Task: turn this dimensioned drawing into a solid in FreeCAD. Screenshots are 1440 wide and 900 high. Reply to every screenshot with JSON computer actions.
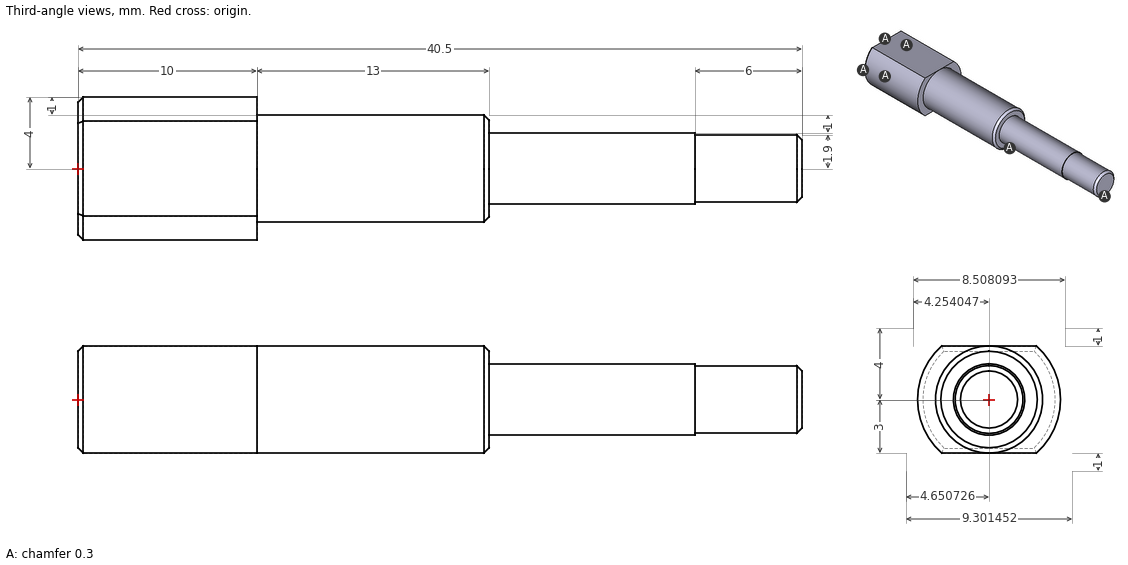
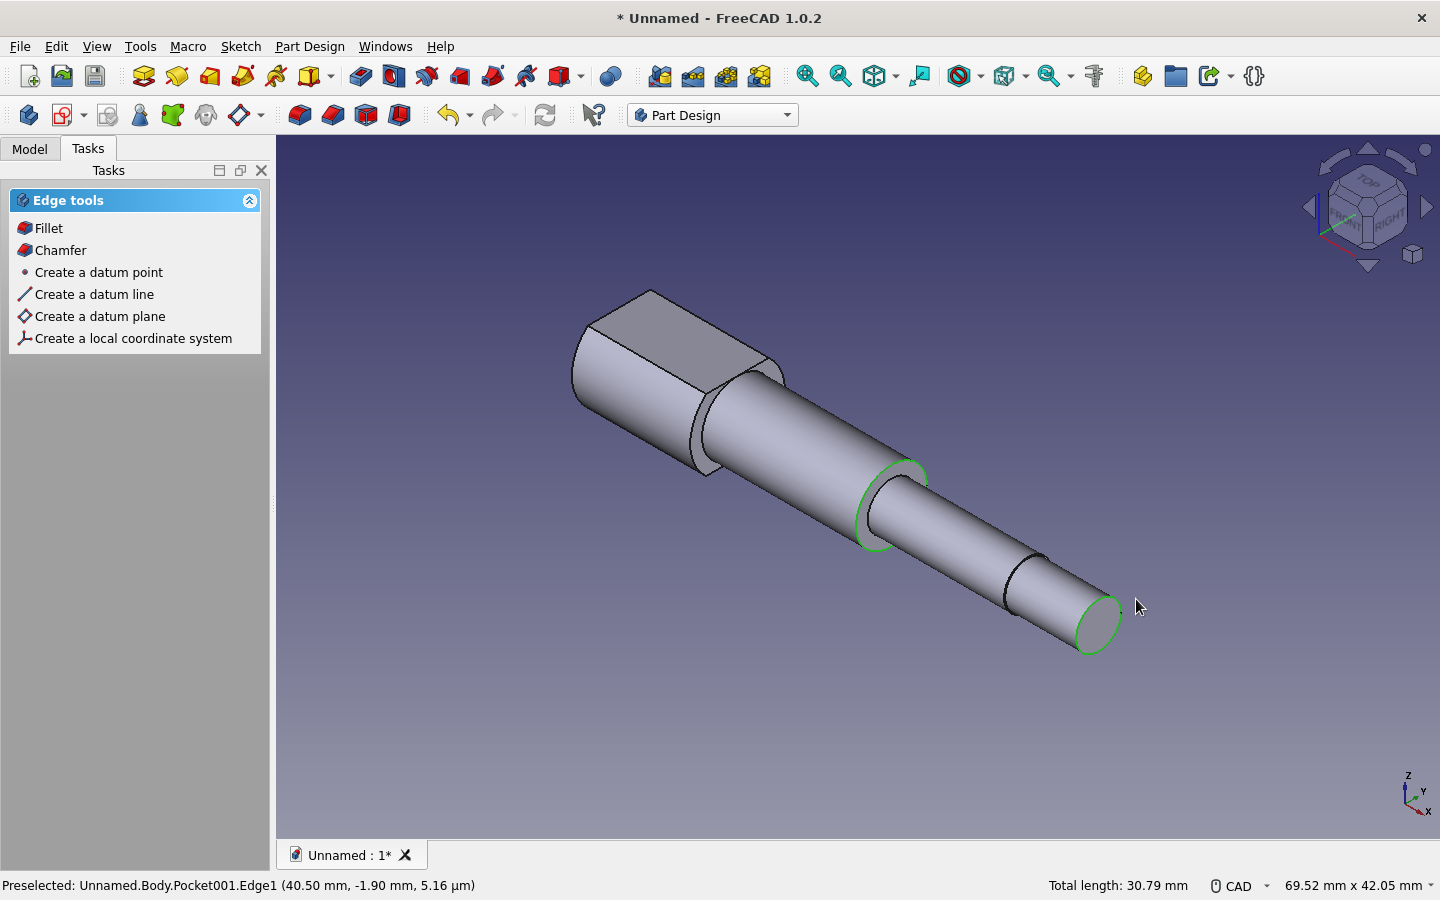
{"action": "left_click", "coordinate": [574, 392], "text": "ctrl"}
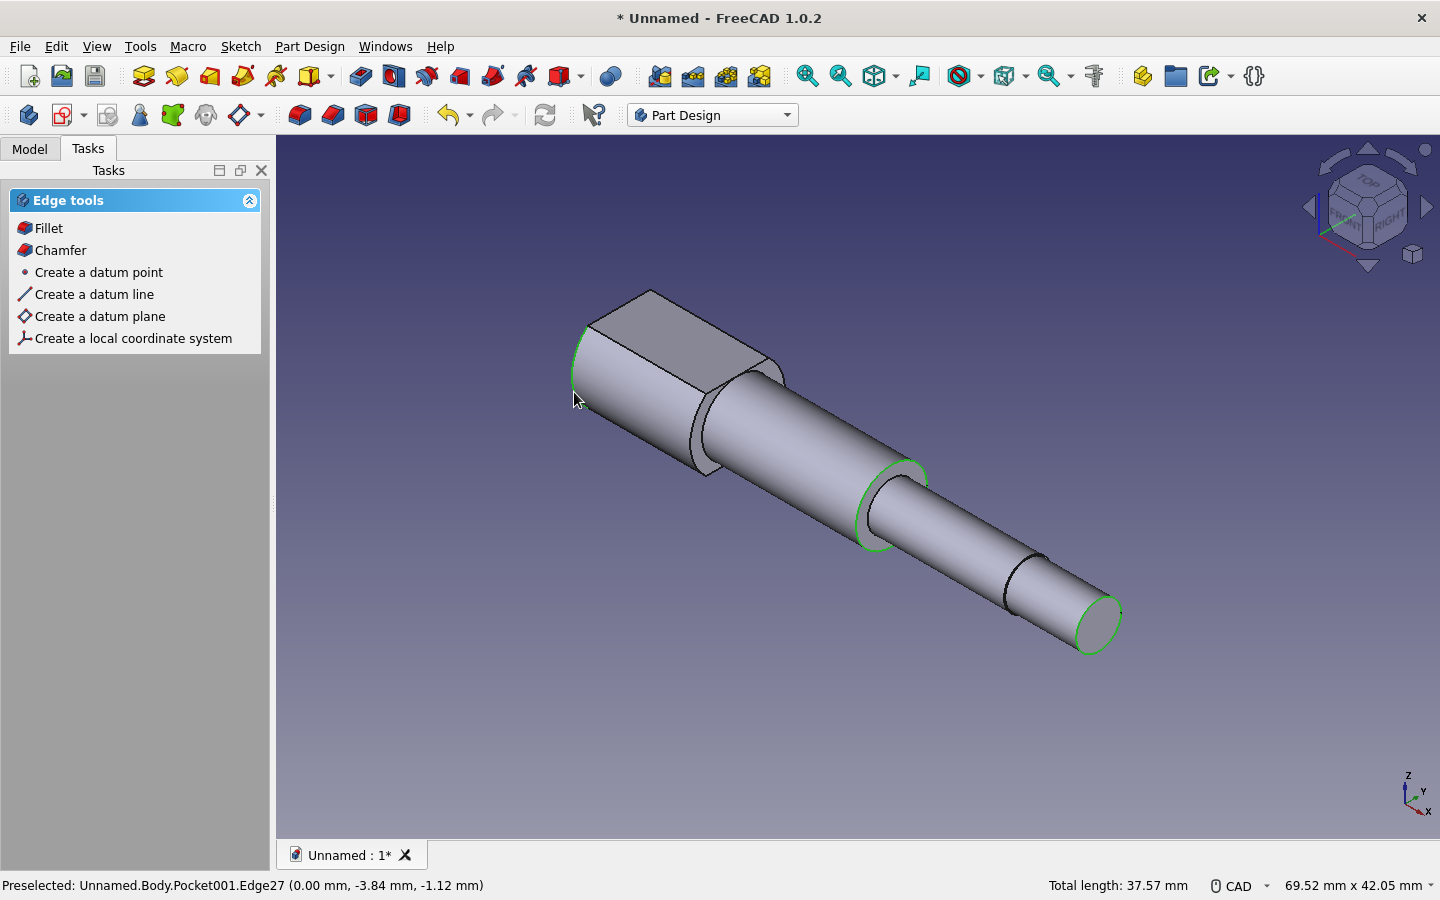
{"action": "key", "text": "2"}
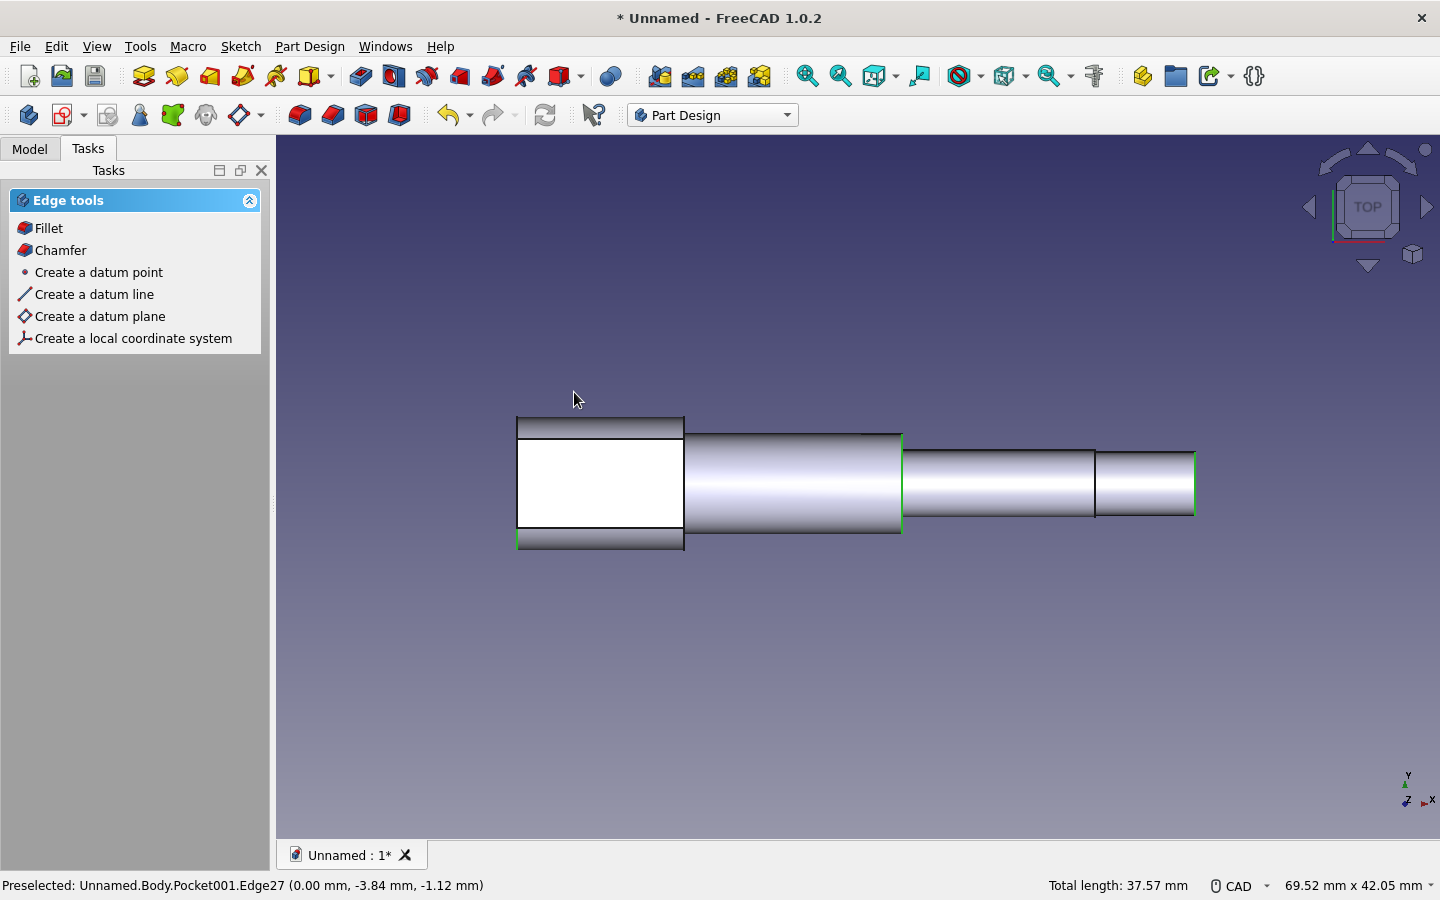
{"action": "left_click", "coordinate": [517, 483], "text": "ctrl"}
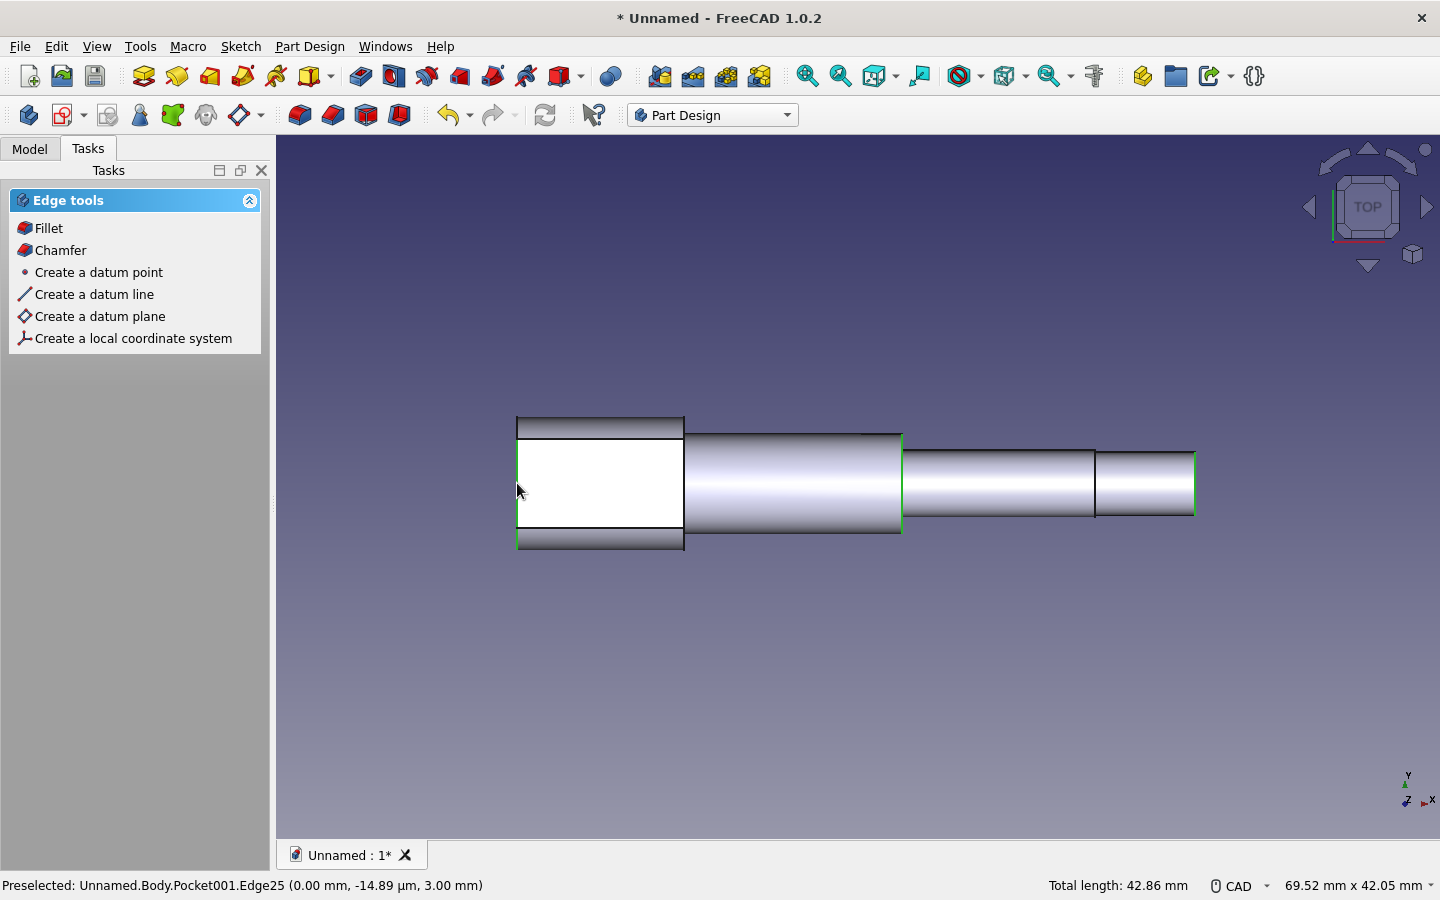
{"action": "key", "text": "1"}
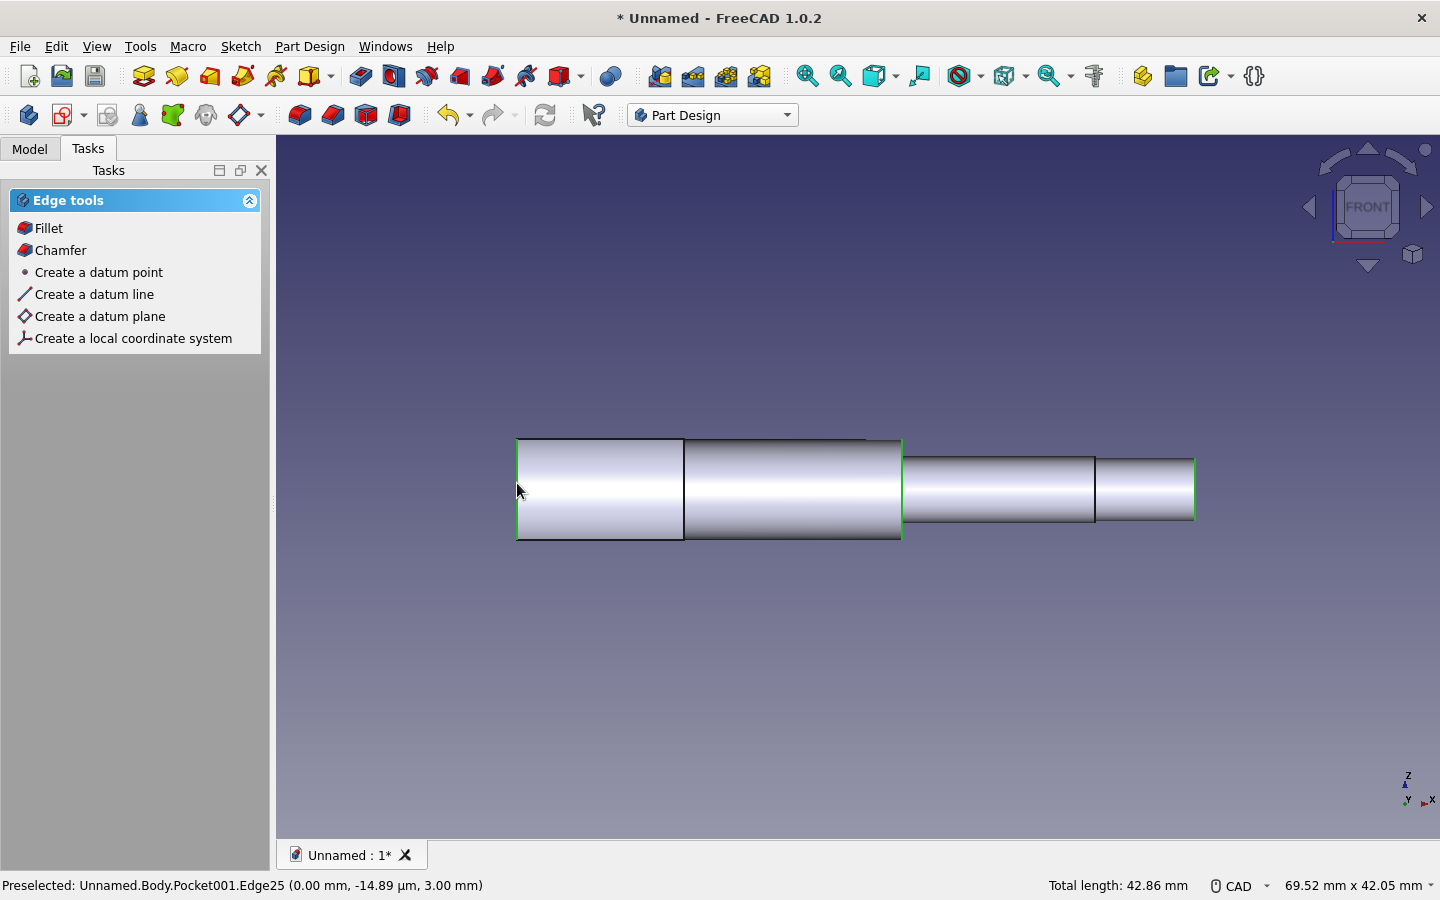
{"action": "key", "text": "3"}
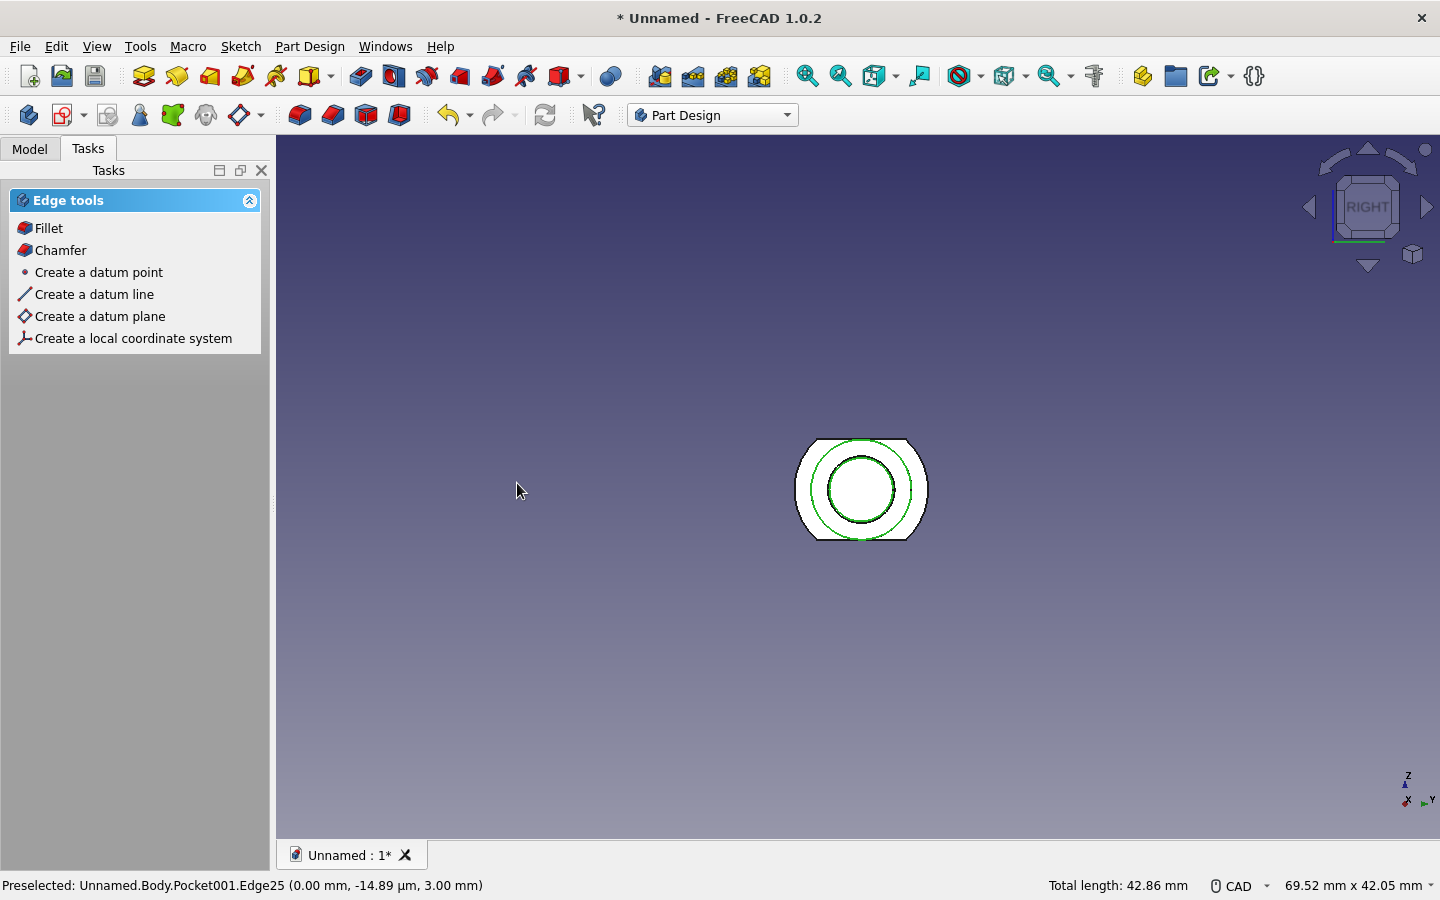
{"action": "key", "text": "v f"}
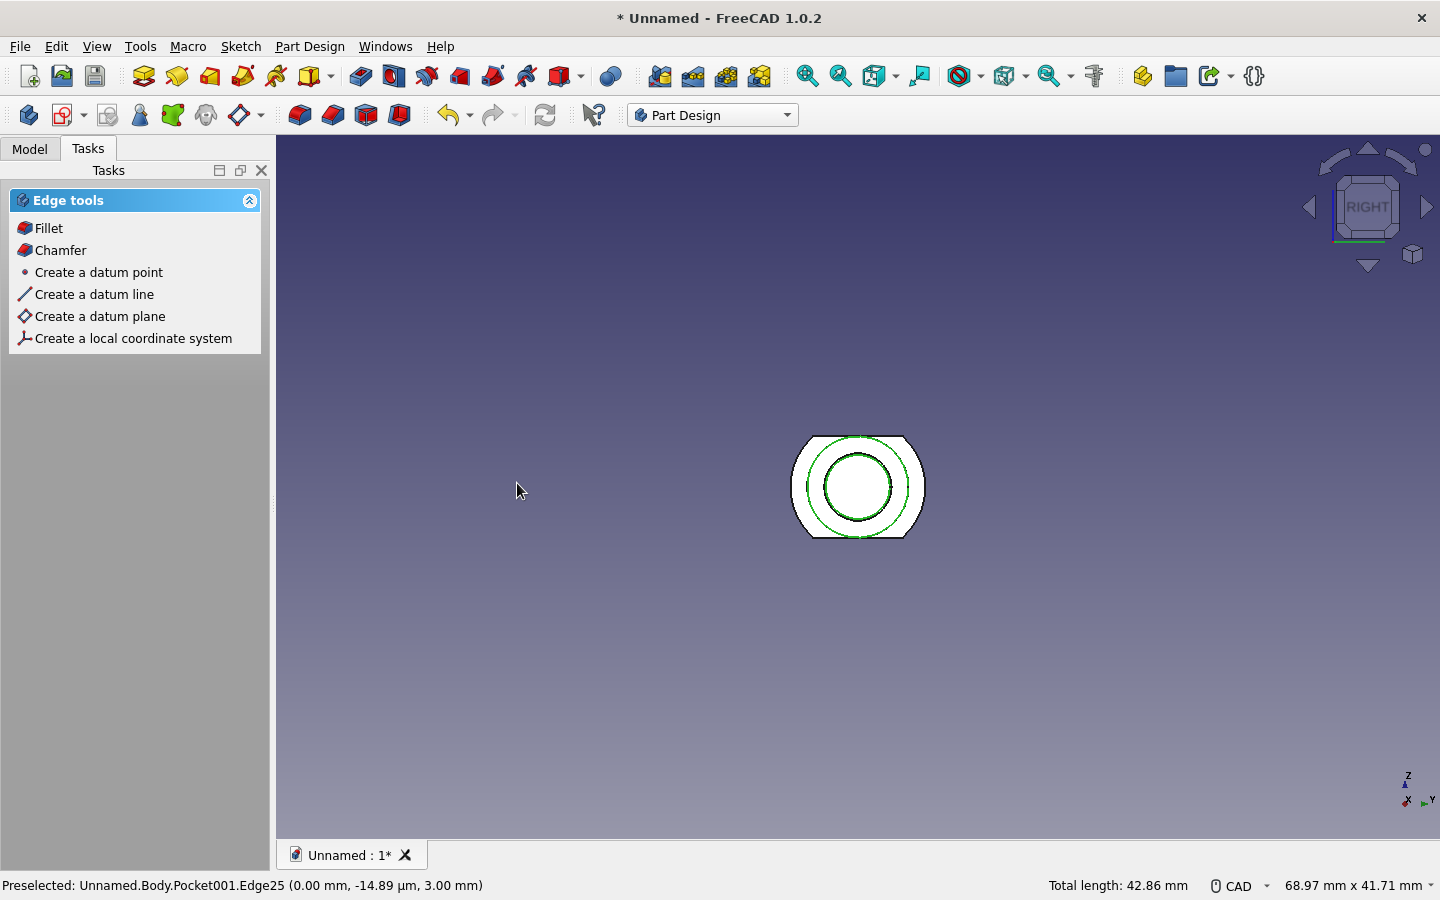
{"action": "key", "text": "5"}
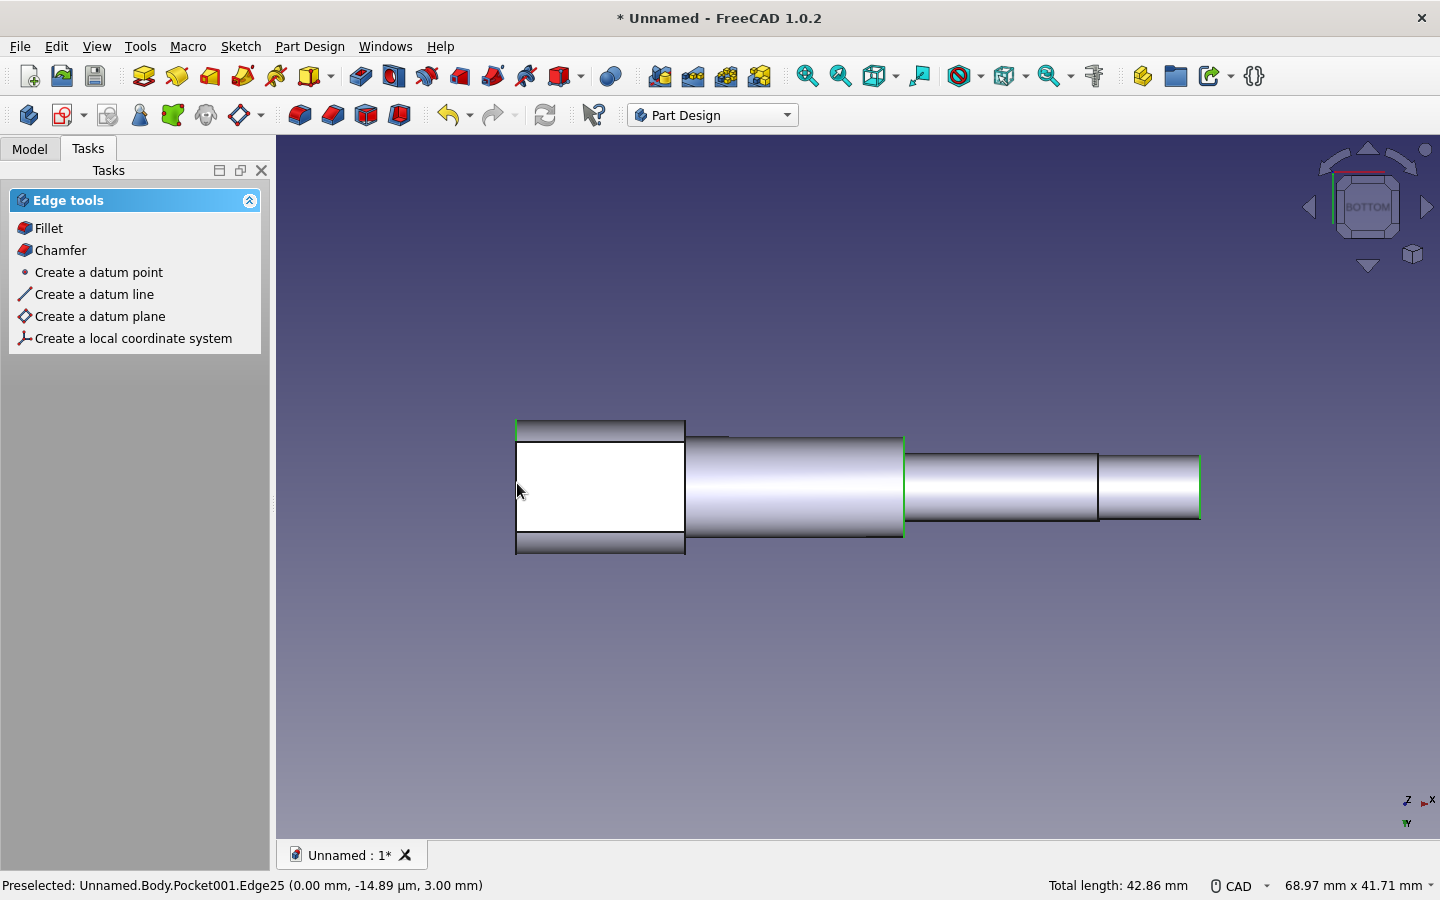
{"action": "left_click", "coordinate": [516, 547], "text": "ctrl"}